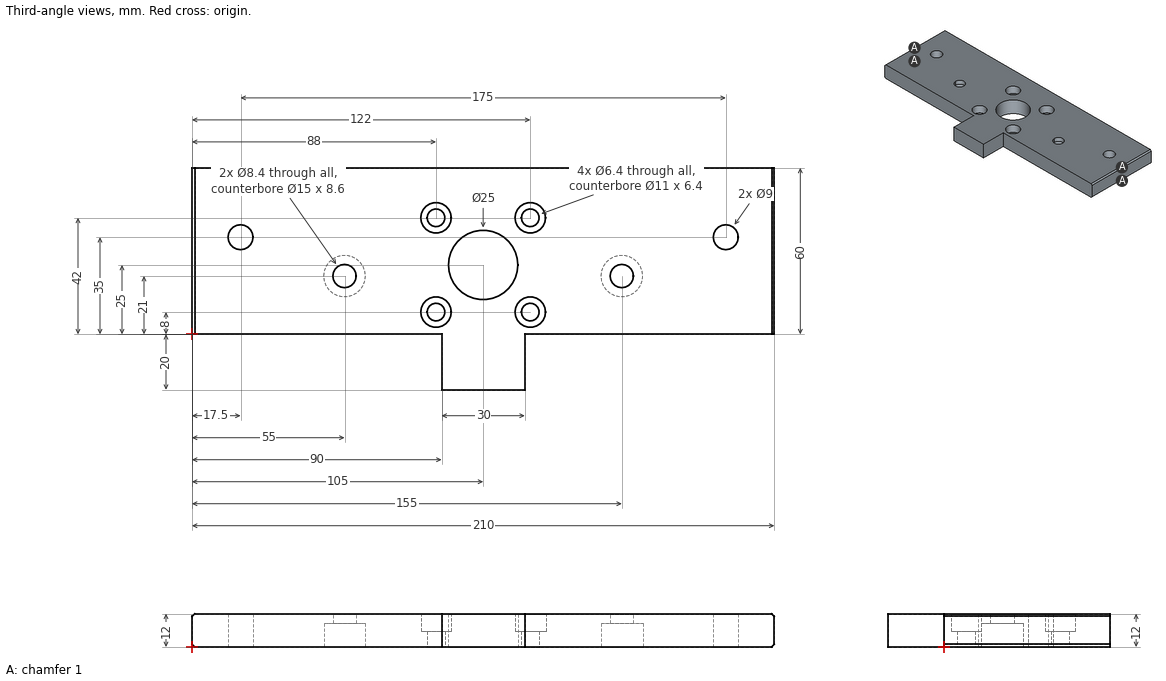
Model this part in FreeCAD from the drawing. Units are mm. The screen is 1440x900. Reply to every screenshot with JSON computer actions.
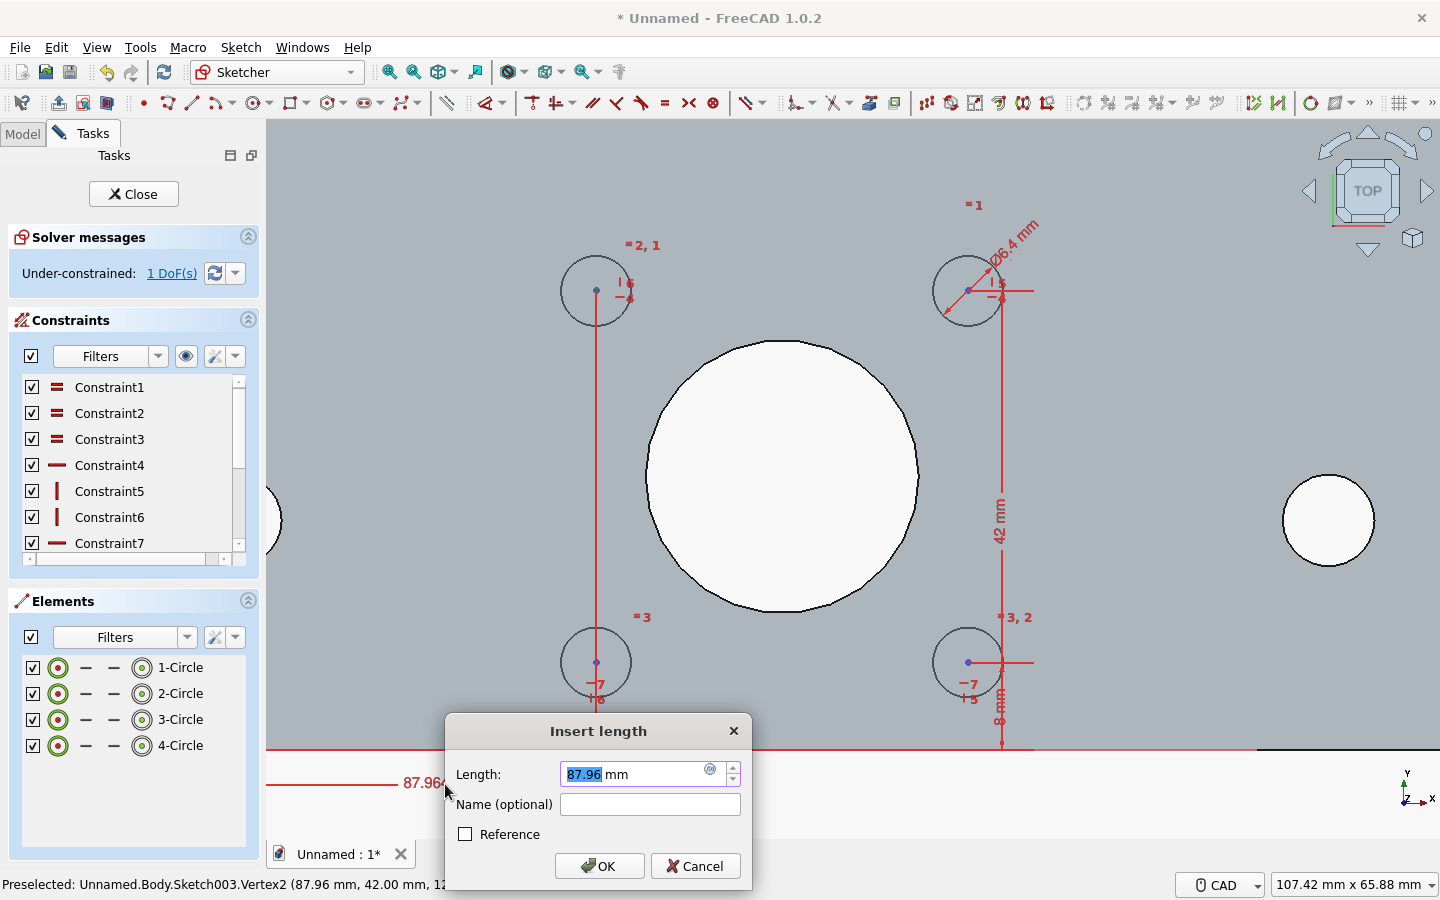
{"action": "type", "text": "88"}
{"action": "key", "text": "Return"}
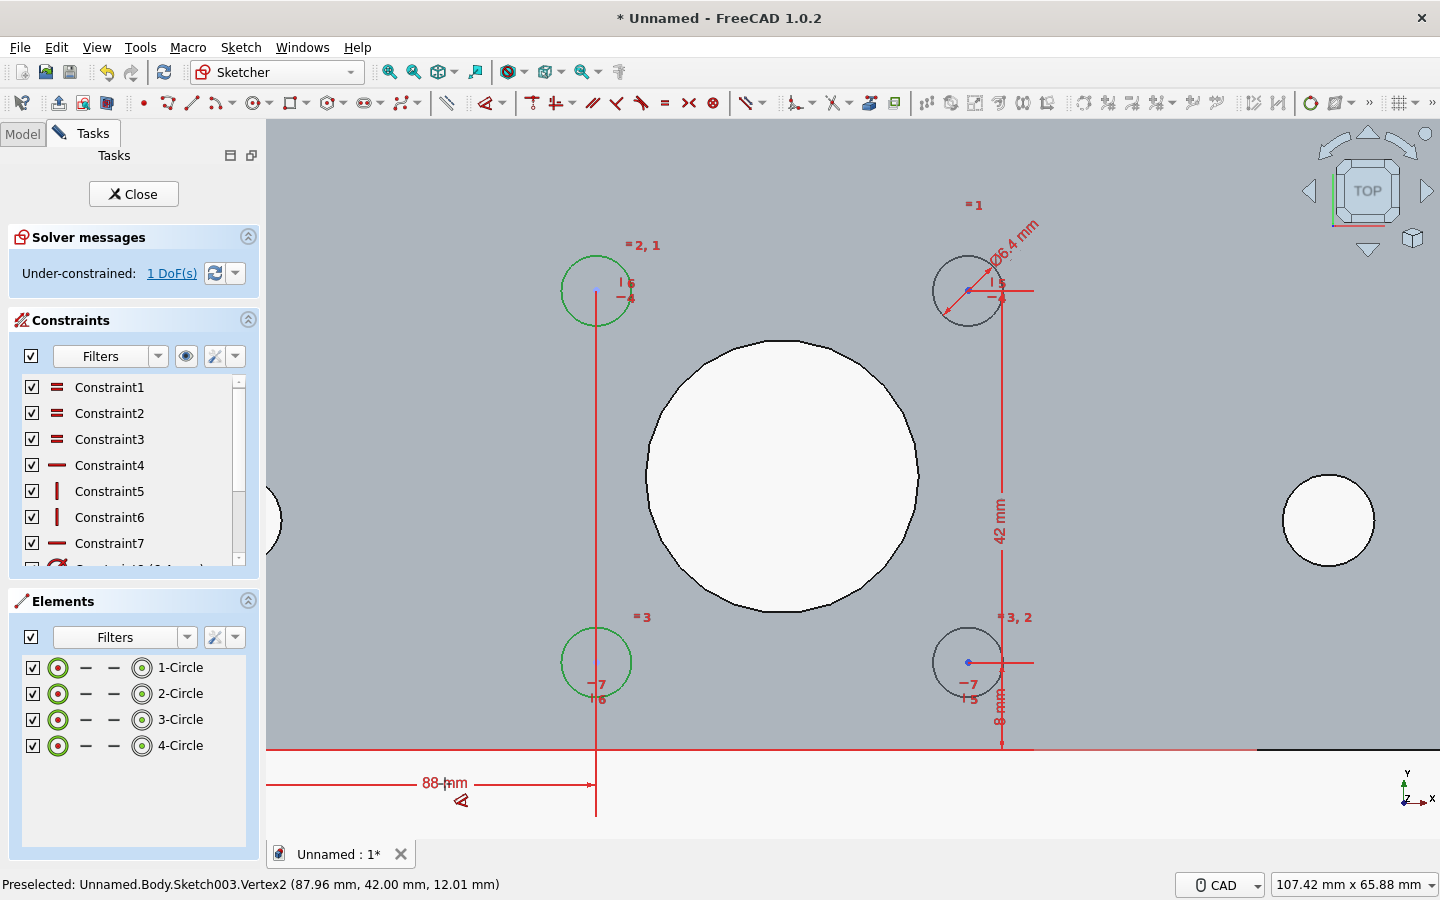
{"action": "left_click", "coordinate": [968, 291]}
{"action": "left_click", "coordinate": [631, 784]}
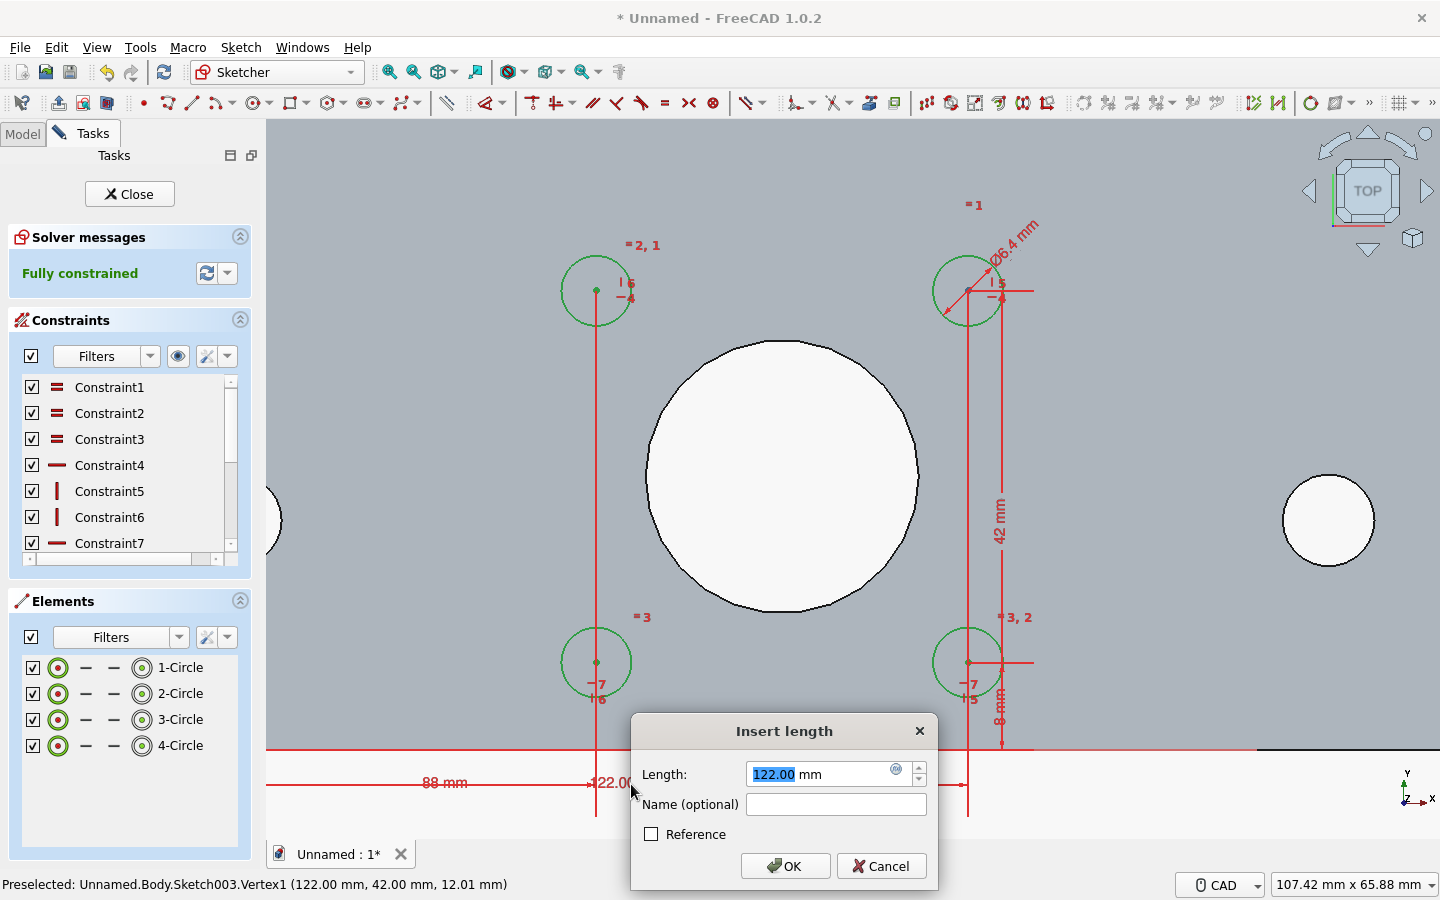
{"action": "type", "text": "122"}
{"action": "key", "text": "Return"}
{"action": "key", "text": "Escape"}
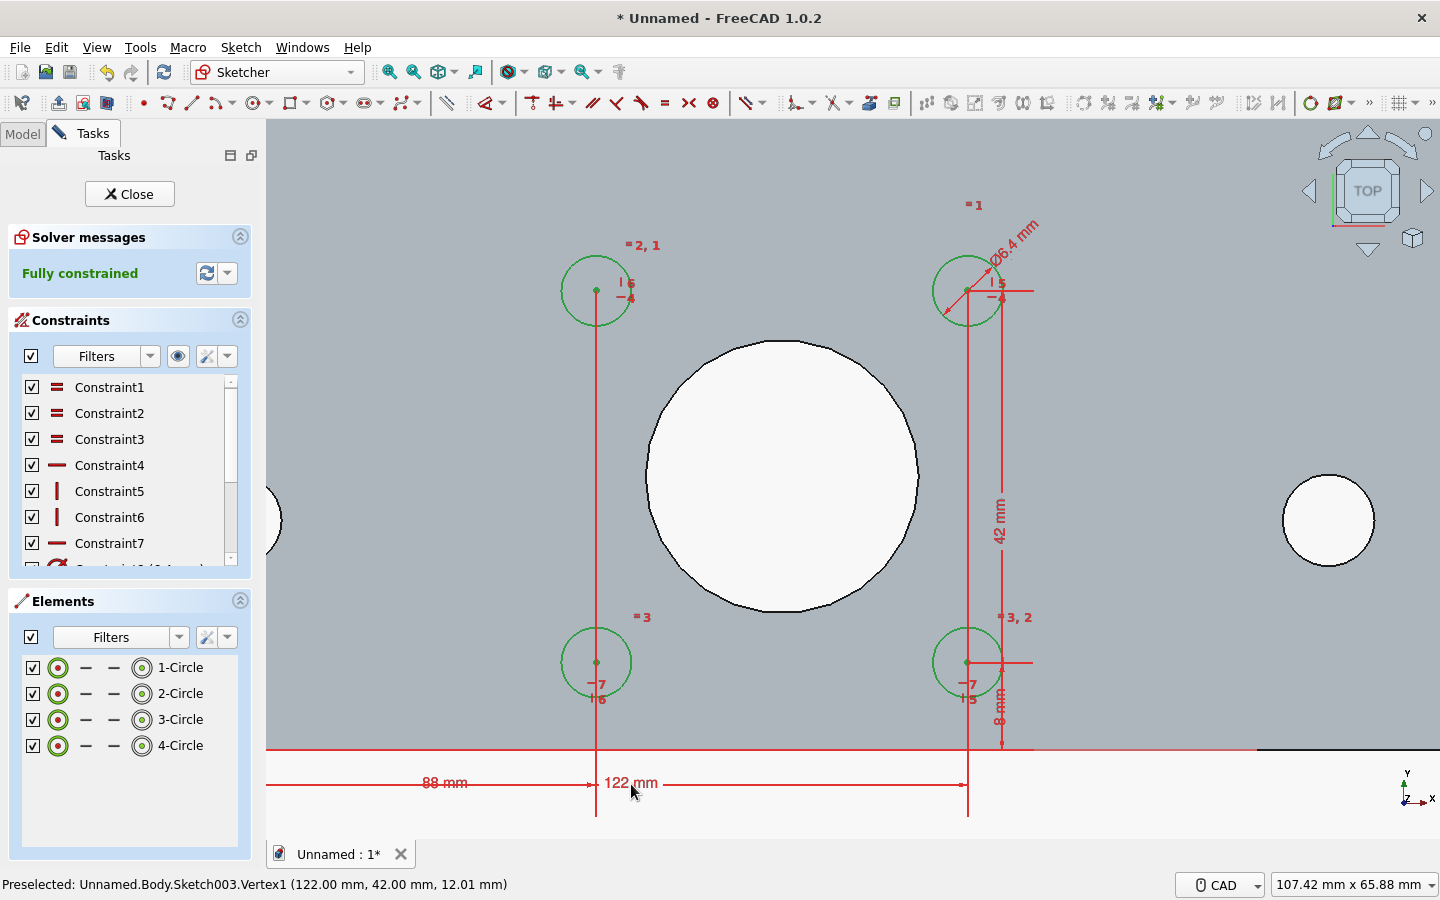
{"action": "left_click", "coordinate": [130, 194]}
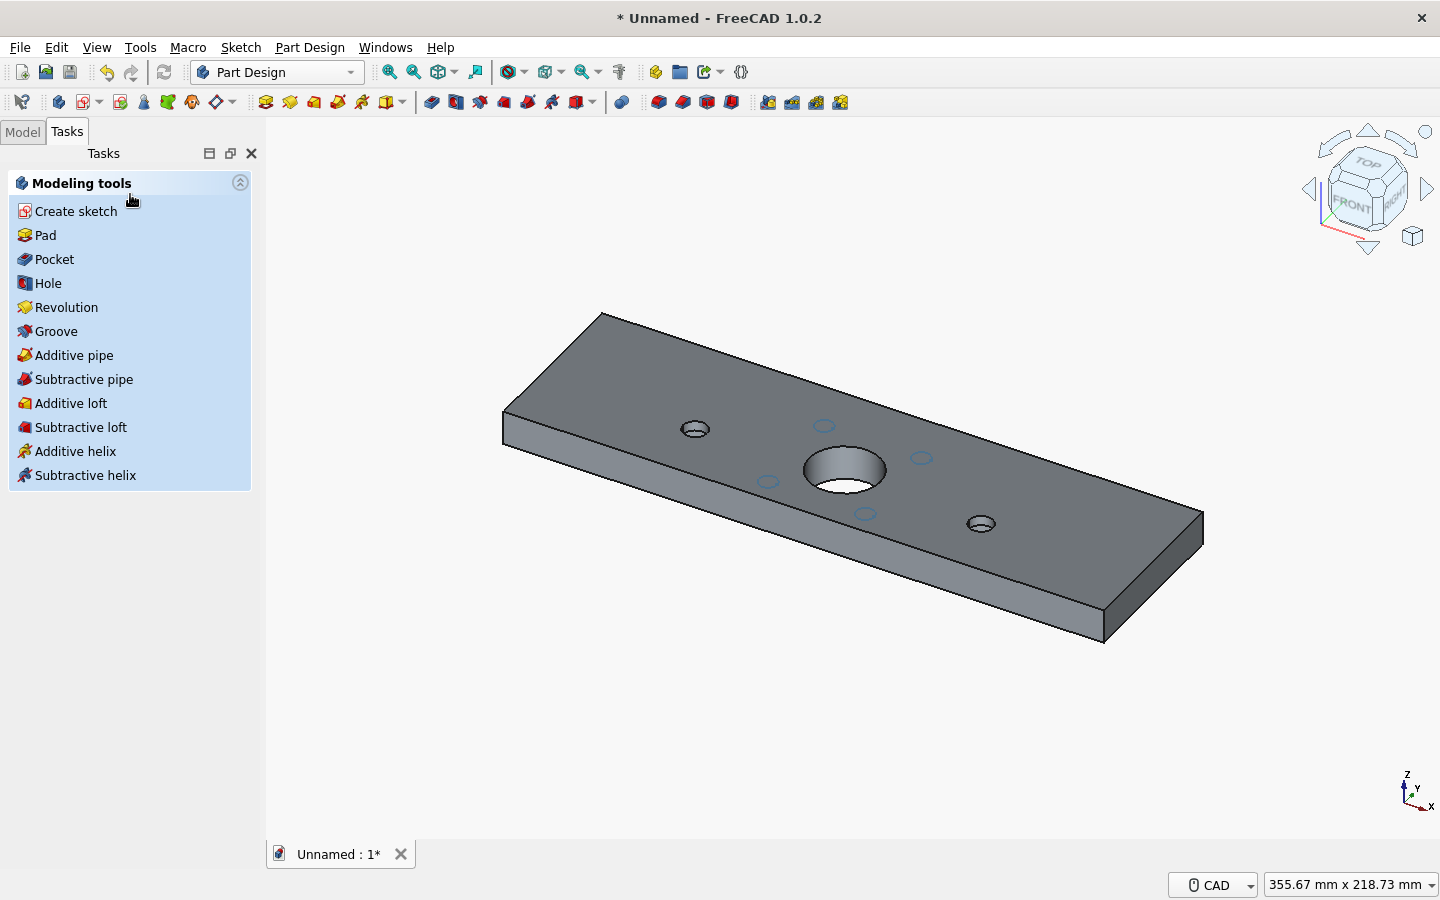
{"action": "left_click", "coordinate": [456, 102]}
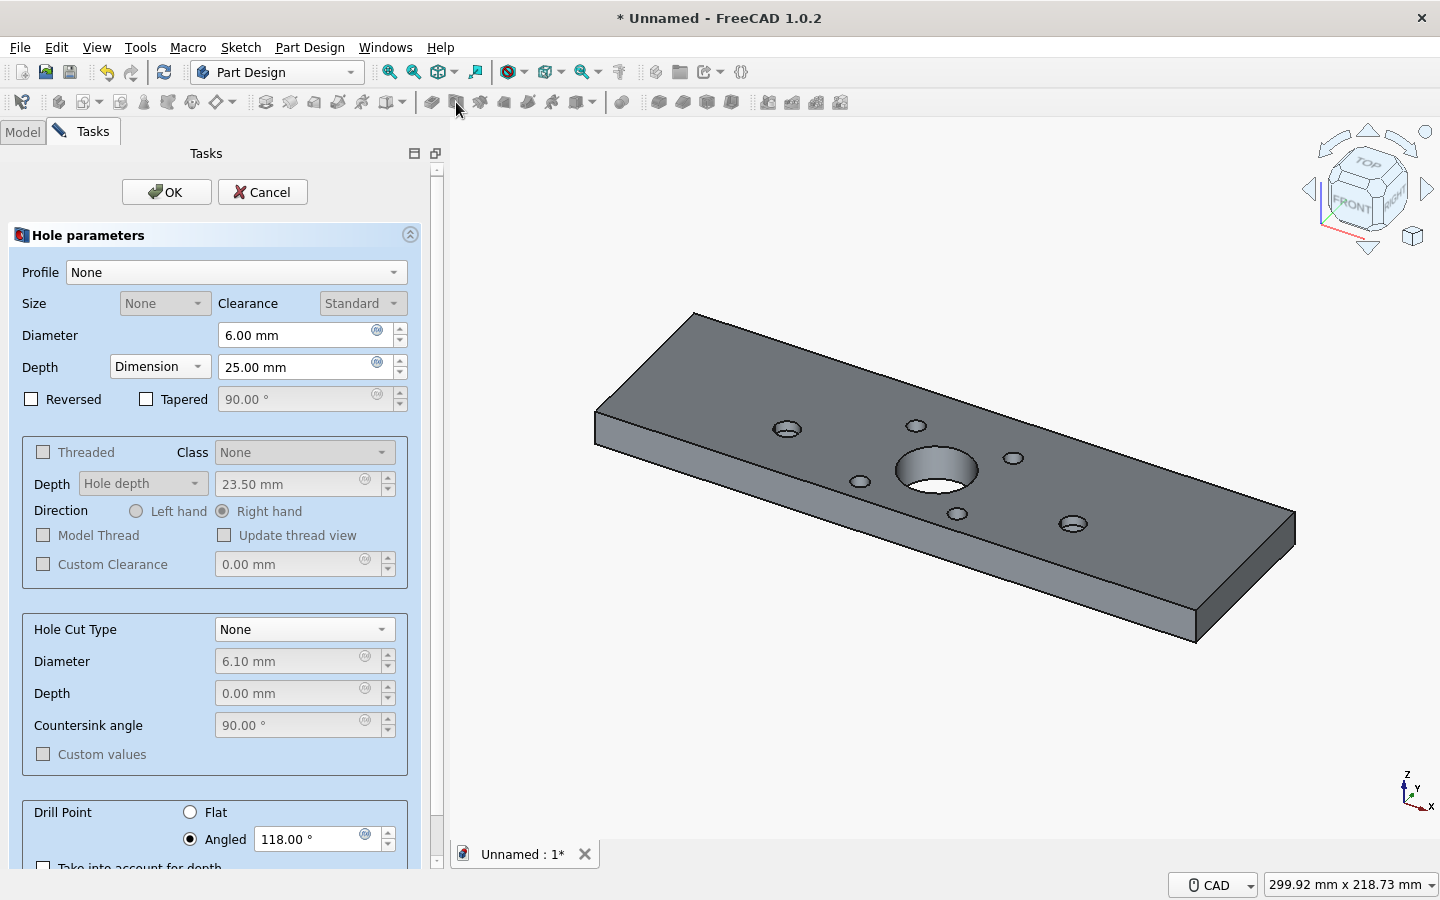
{"action": "triple_click", "coordinate": [305, 335]}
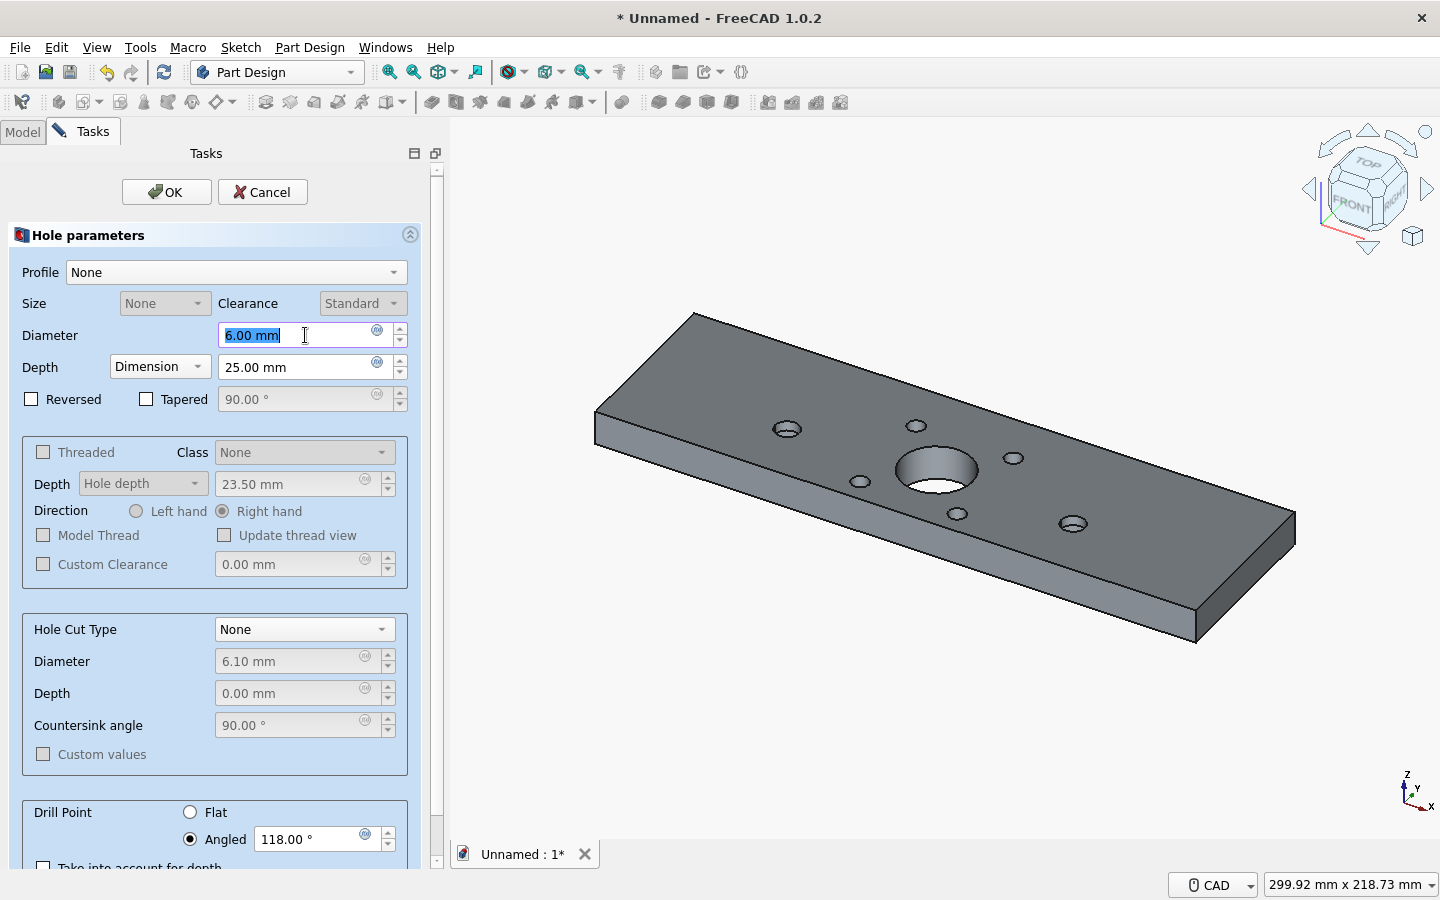
{"action": "type", "text": "6.4"}
{"action": "key", "text": "Tab"}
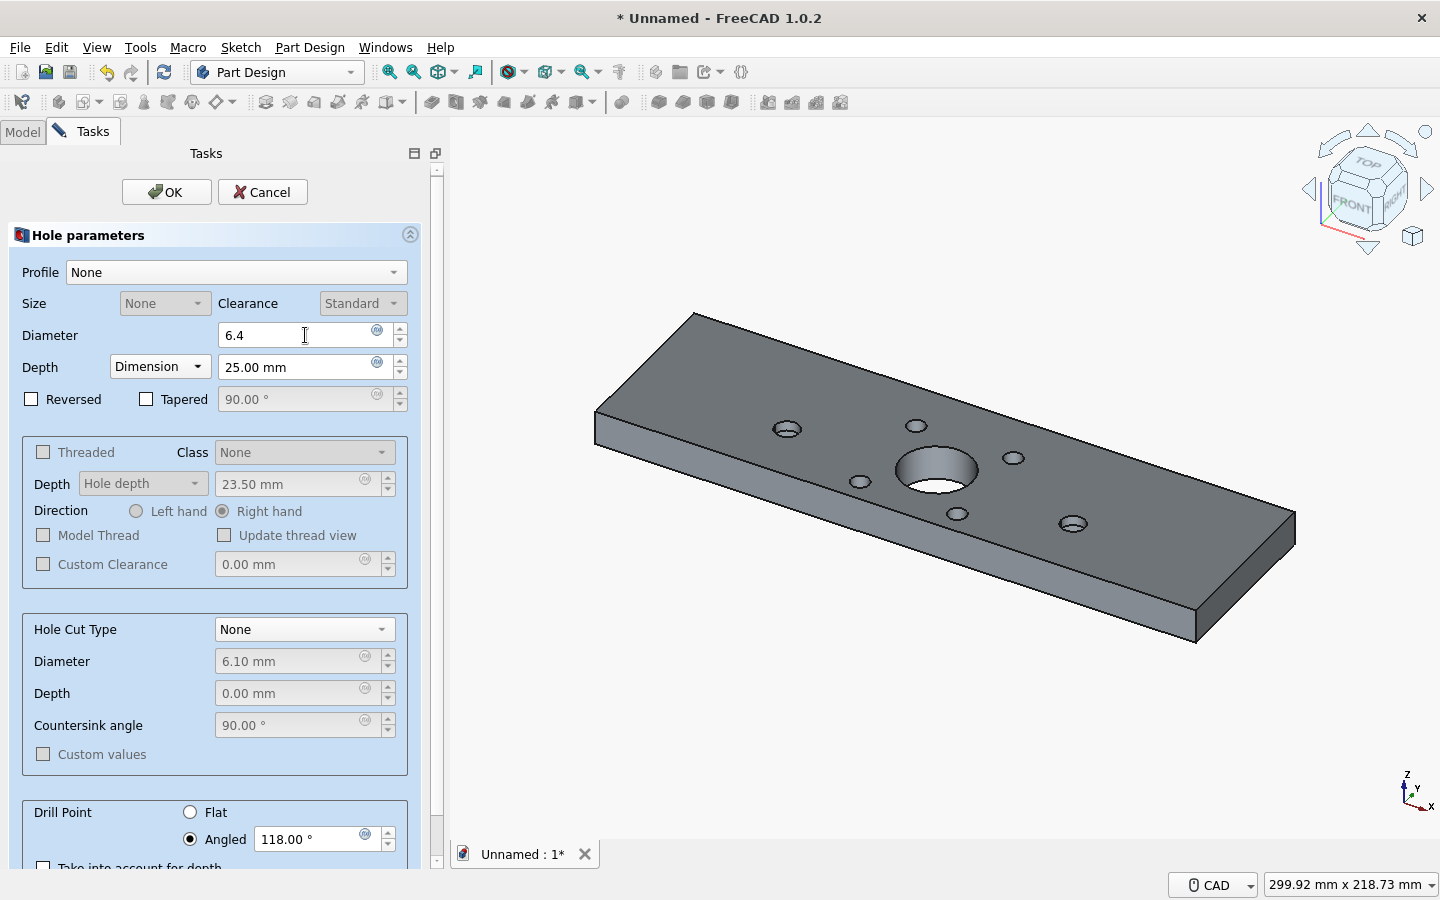
{"action": "left_click", "coordinate": [161, 366]}